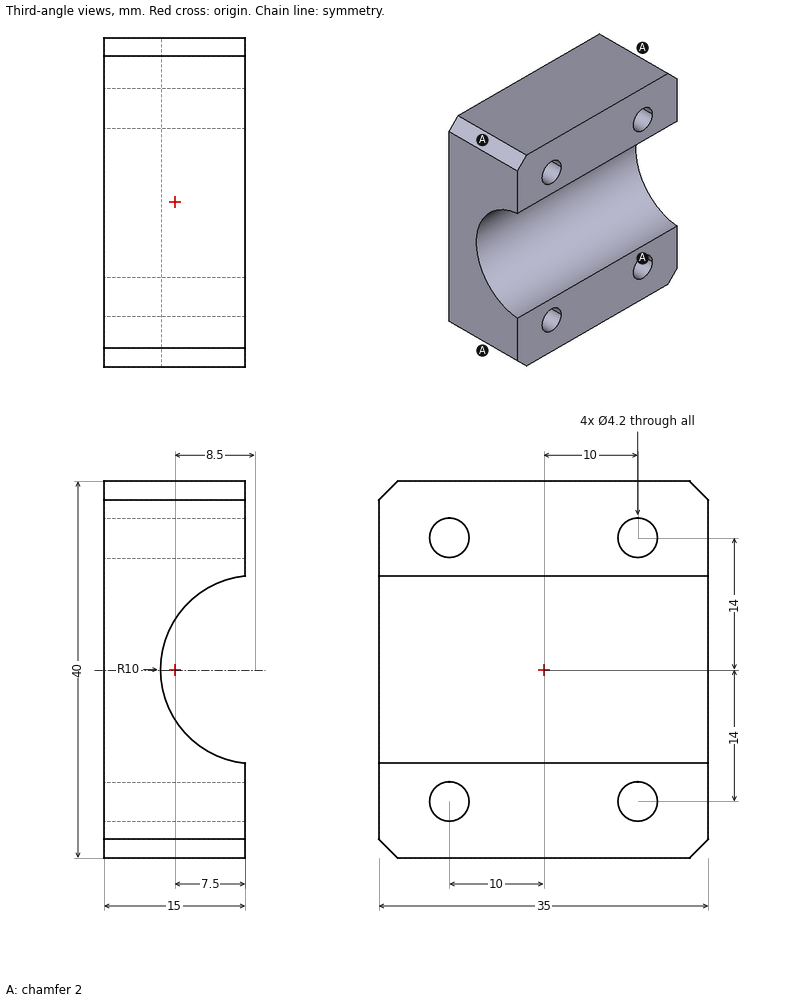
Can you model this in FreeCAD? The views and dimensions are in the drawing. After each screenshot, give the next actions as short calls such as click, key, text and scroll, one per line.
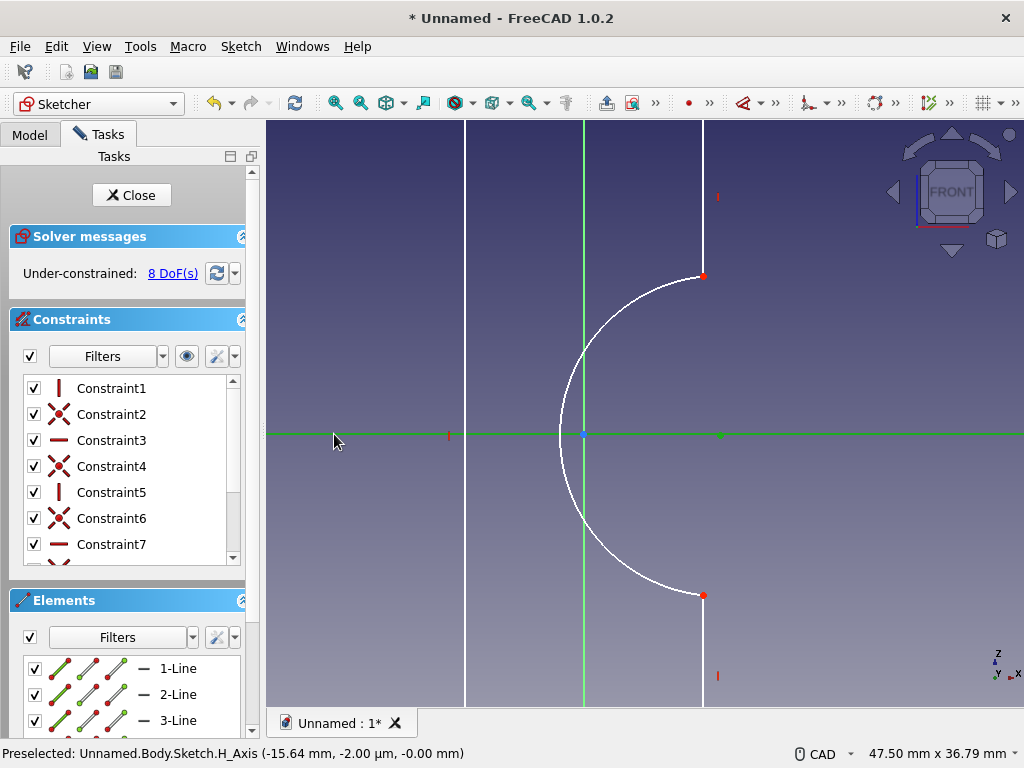
key(c)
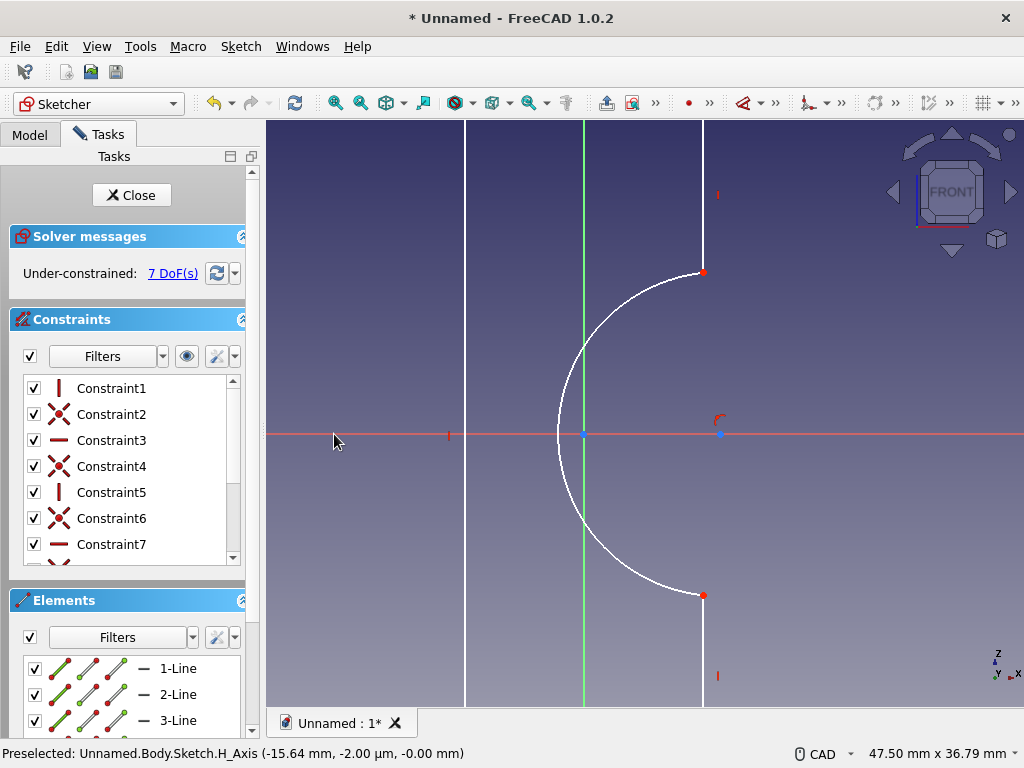
scroll(568, 388, down, 3)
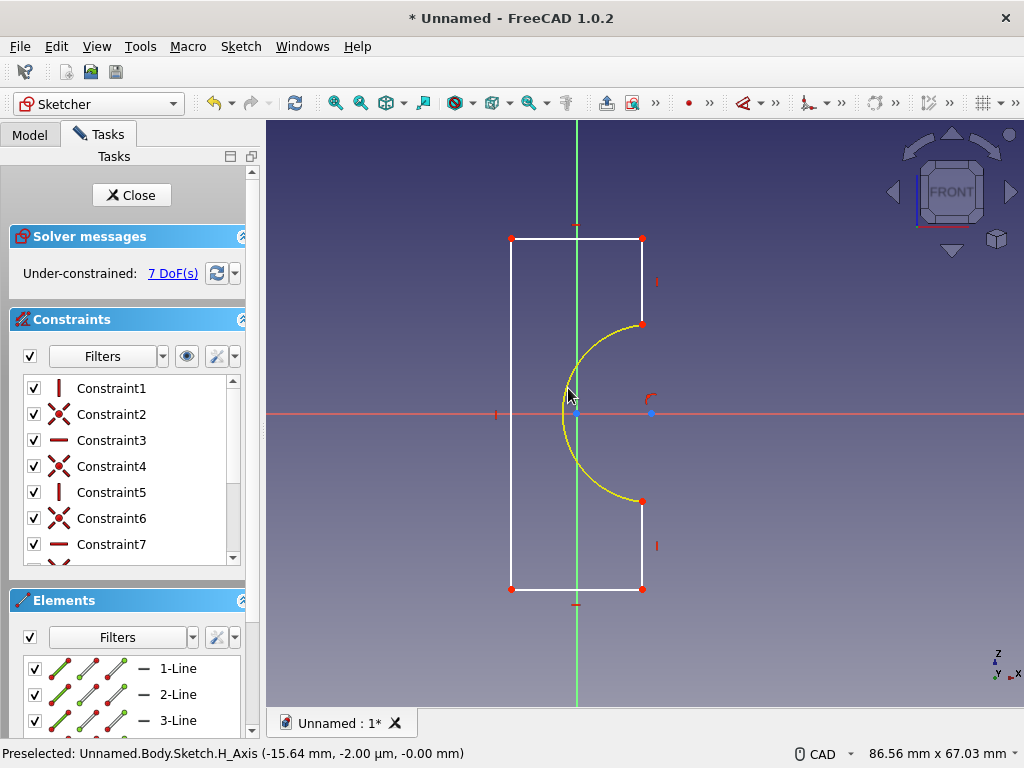
click(642, 590)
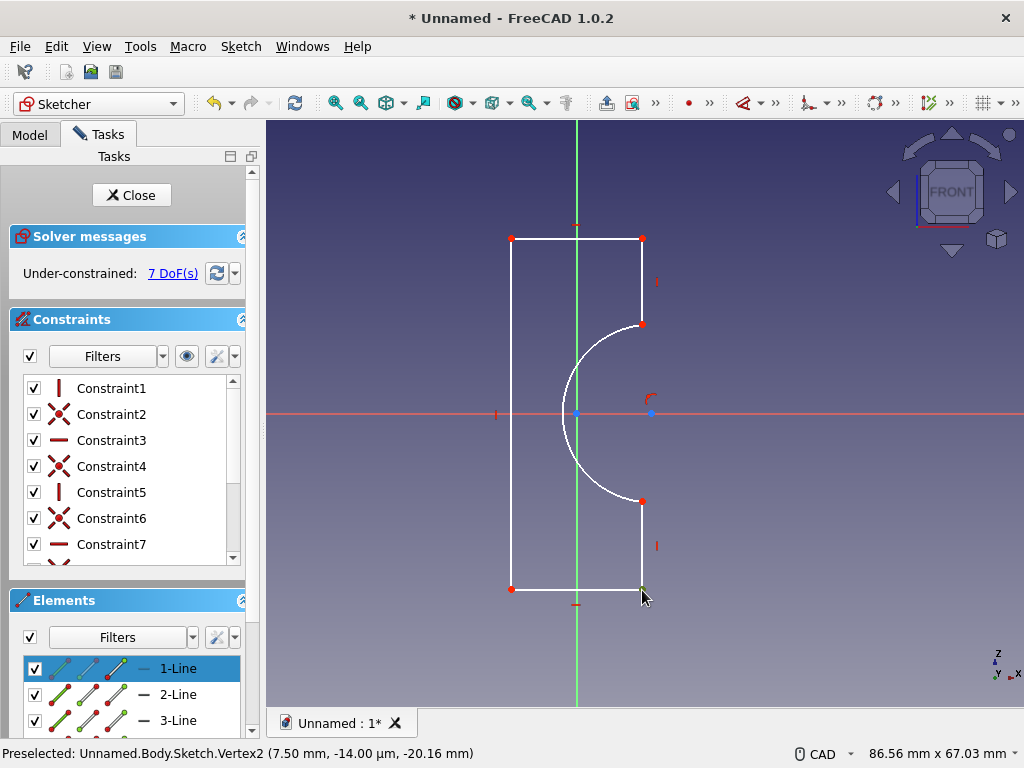
click(642, 239)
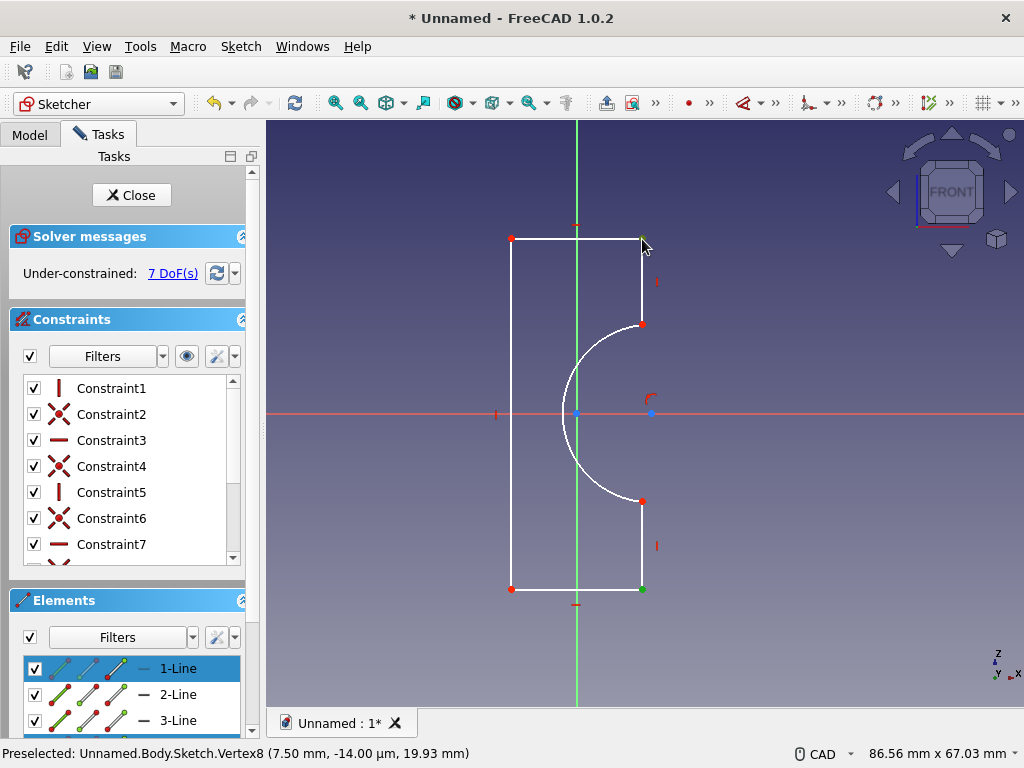
click(334, 413)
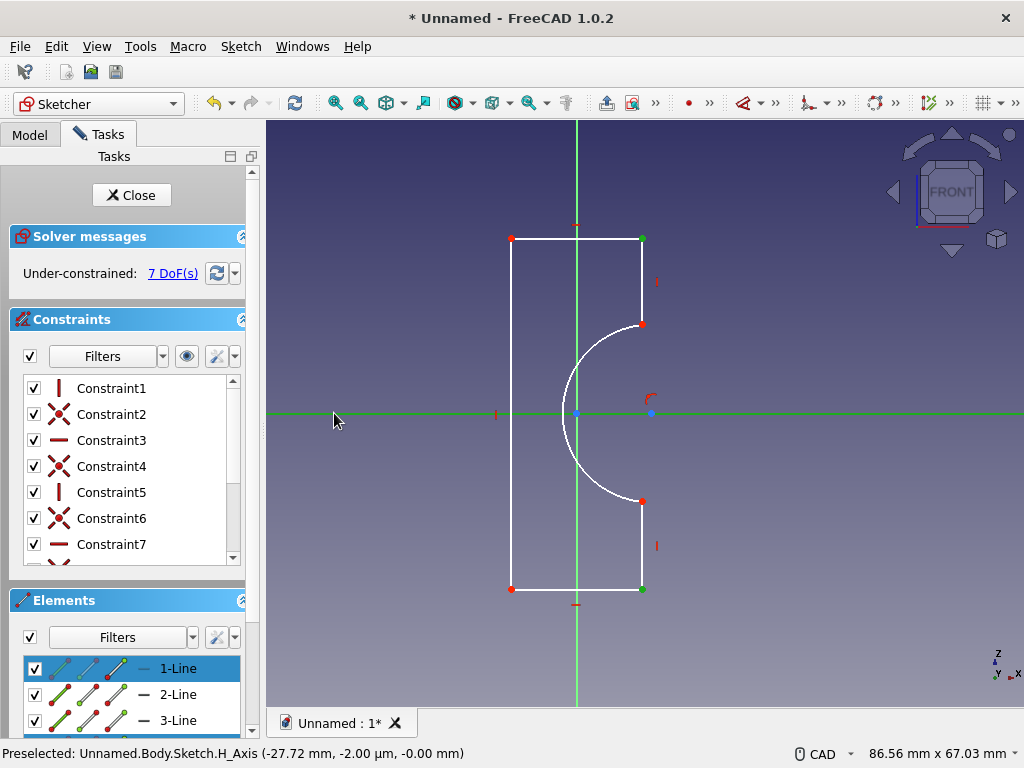
key(s)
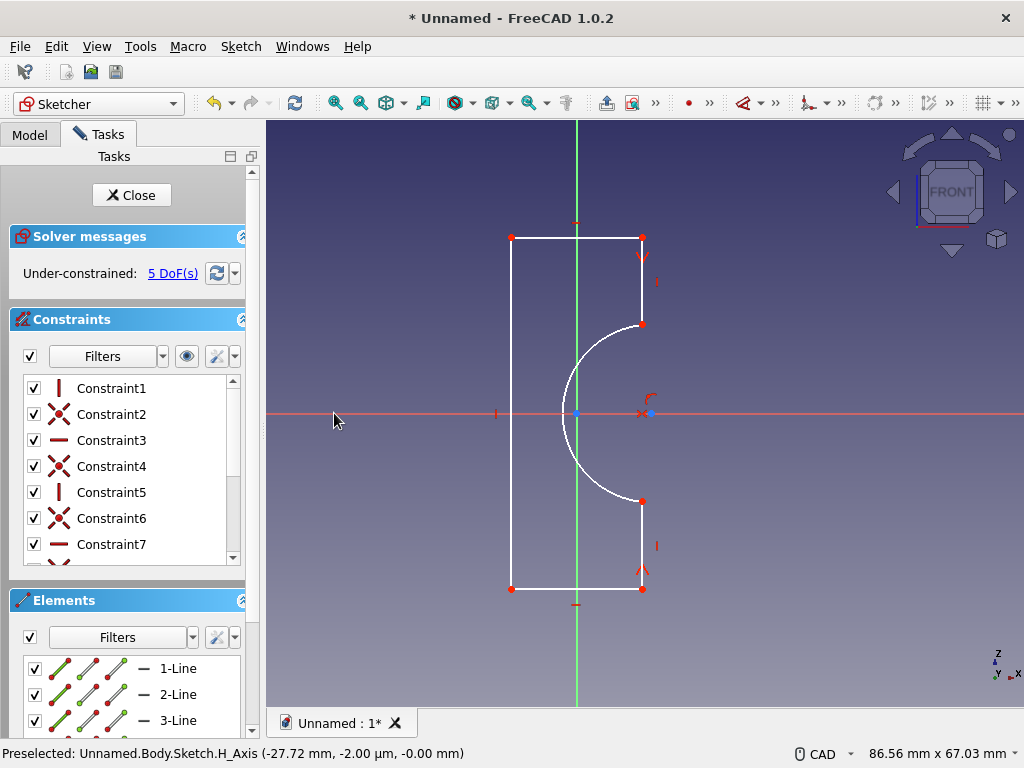
click(742, 104)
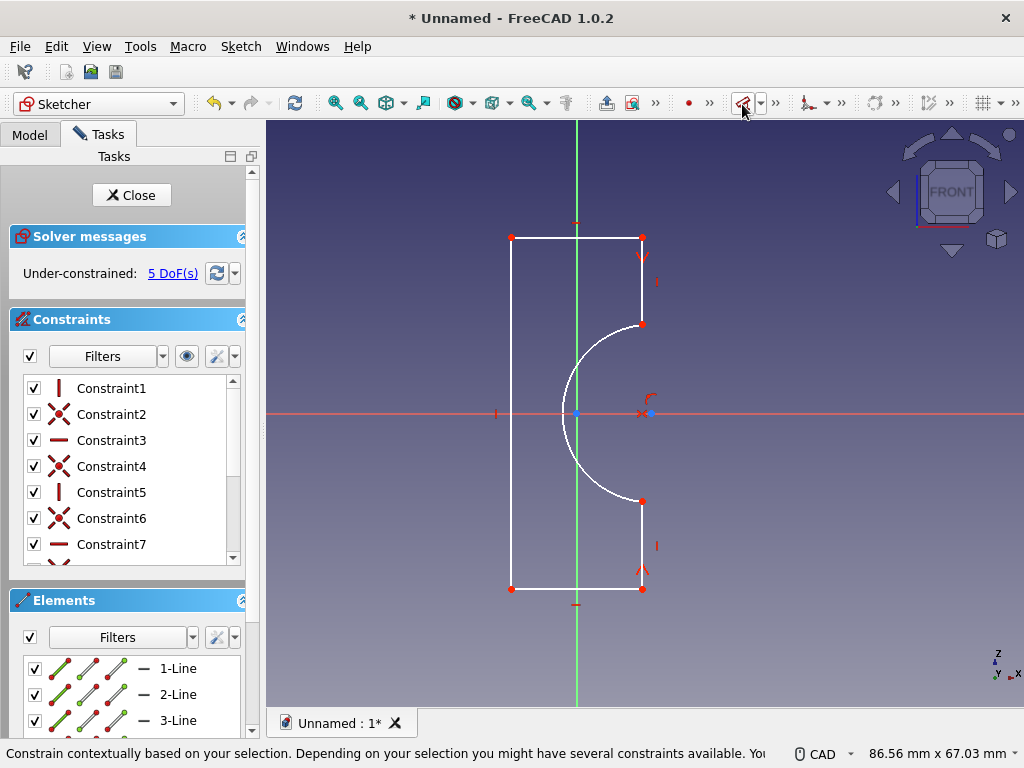
click(578, 364)
click(551, 346)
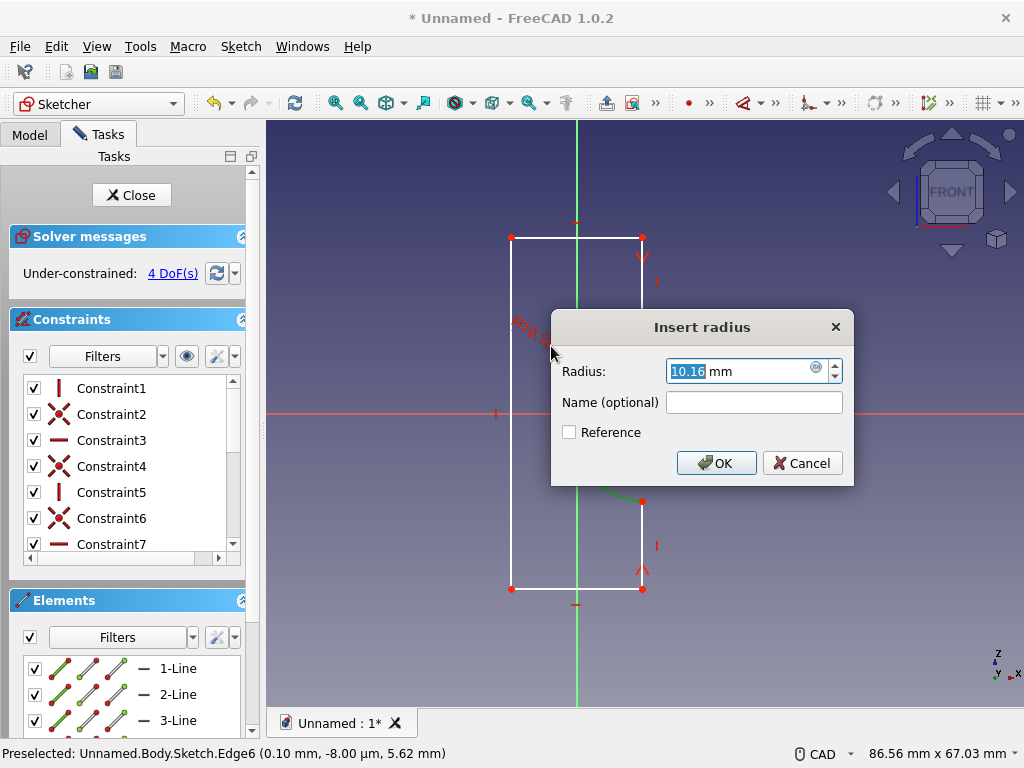
text(10)
key(Return)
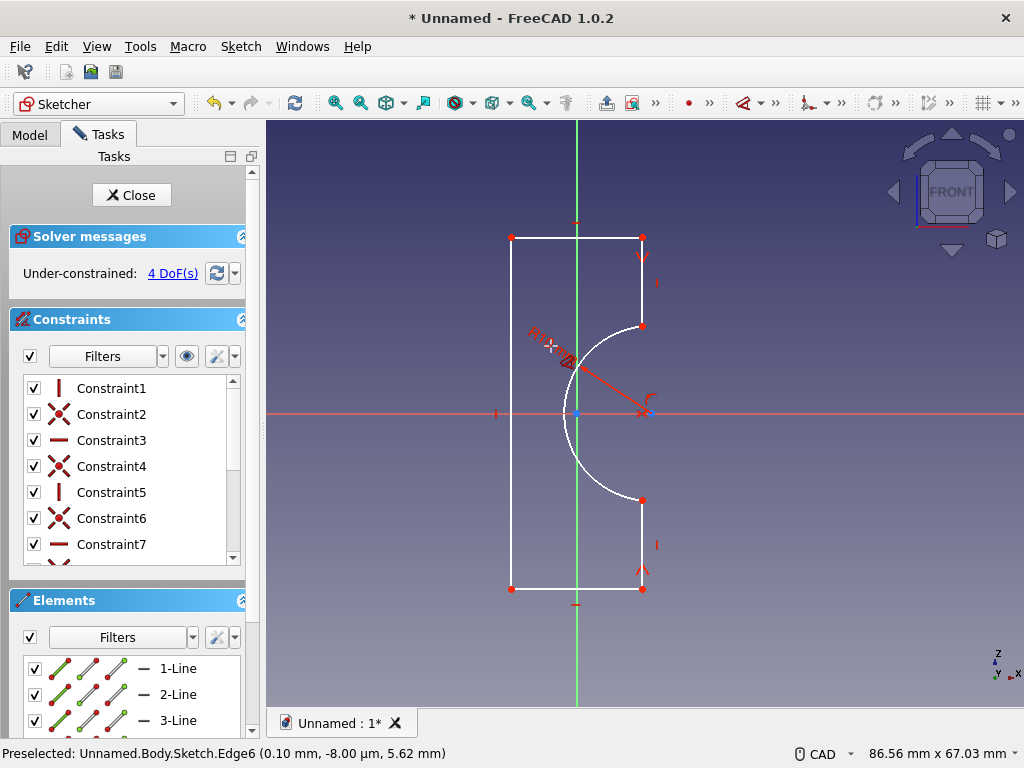
click(603, 589)
click(547, 623)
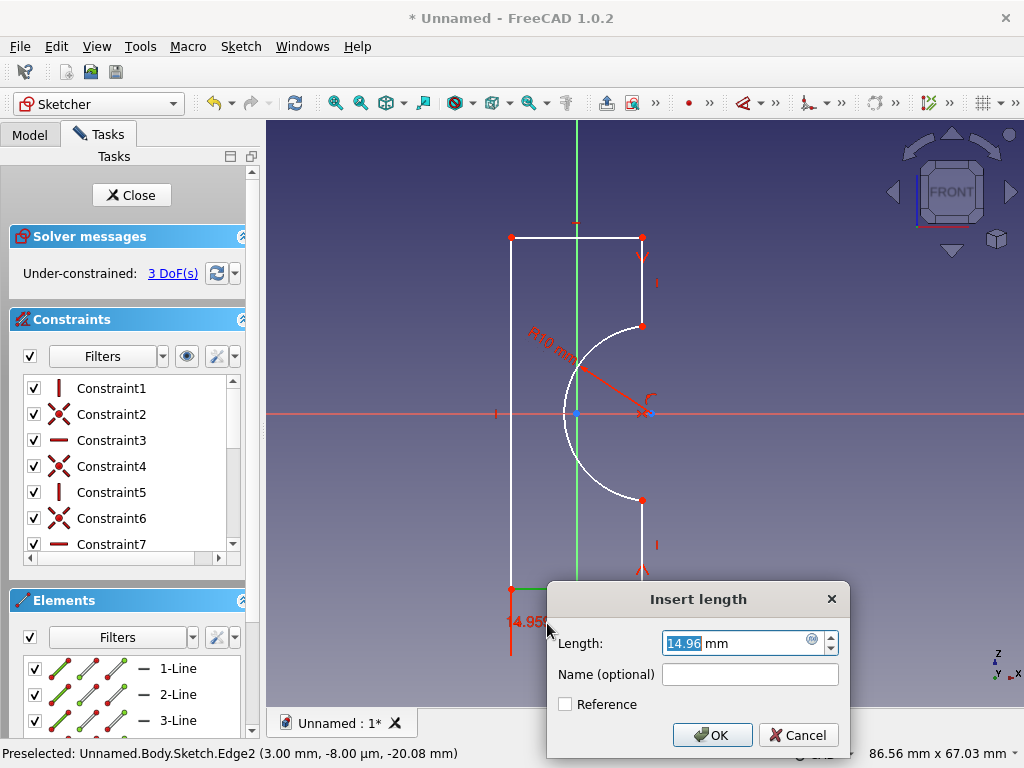
text(15)
key(Return)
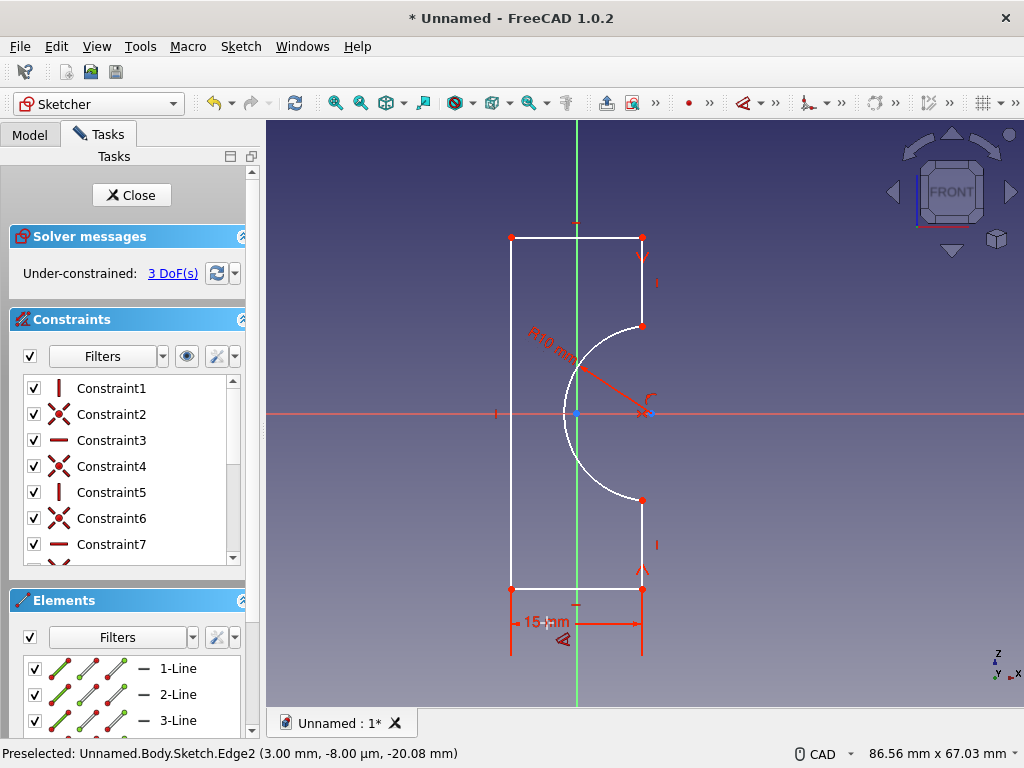
click(511, 484)
click(477, 333)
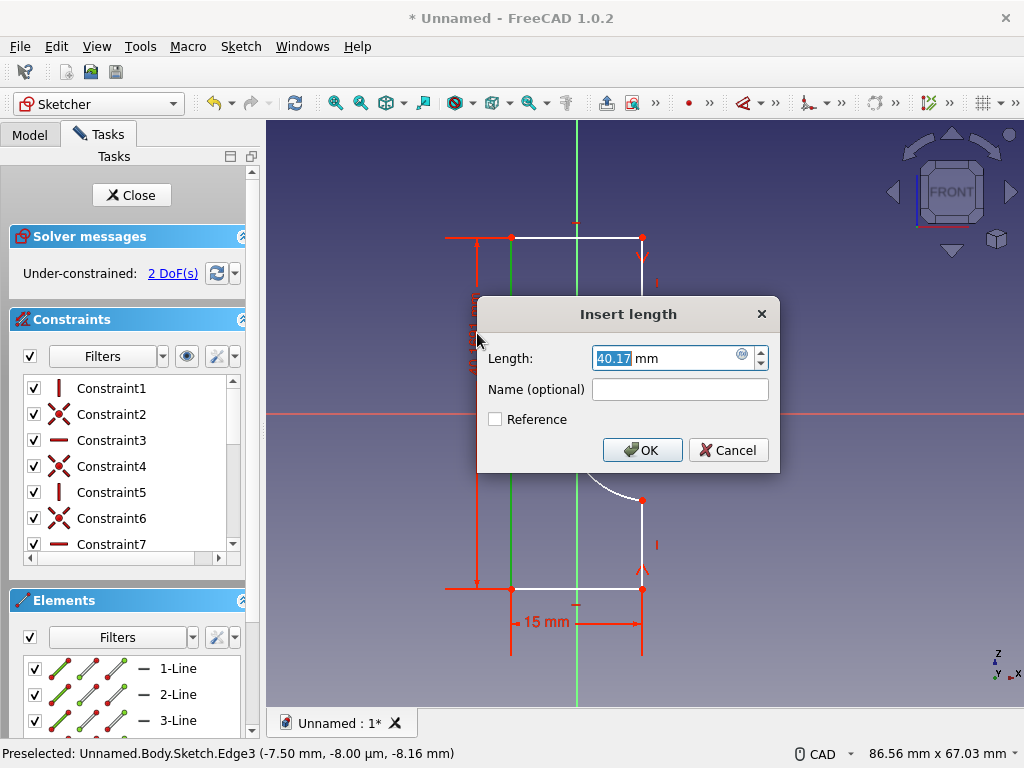
text(40)
key(Return)